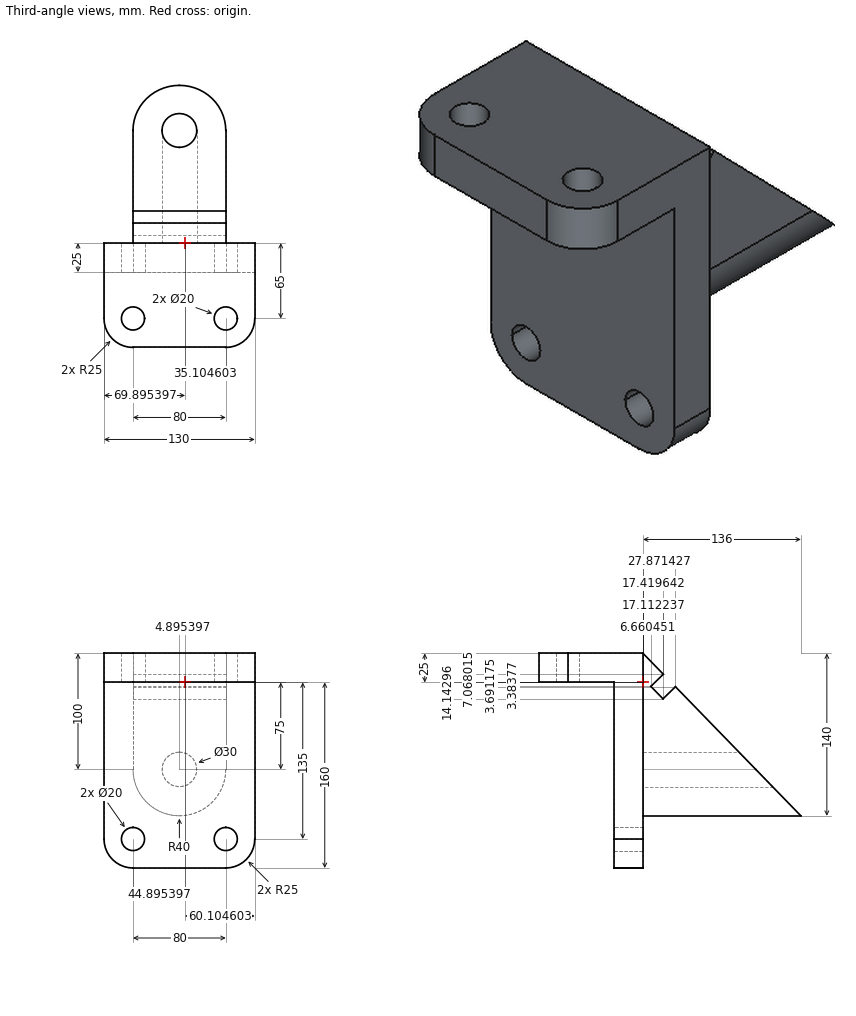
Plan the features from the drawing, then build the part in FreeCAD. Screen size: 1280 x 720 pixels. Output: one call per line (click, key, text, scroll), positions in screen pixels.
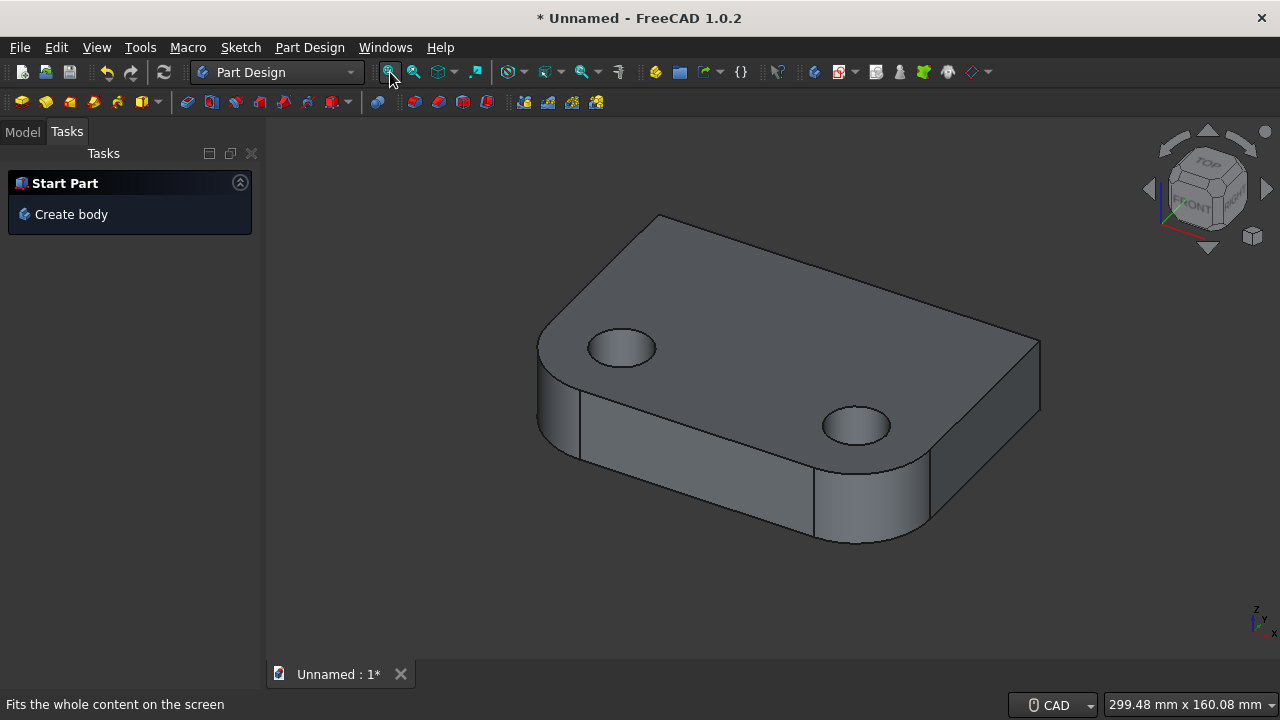
click(840, 72)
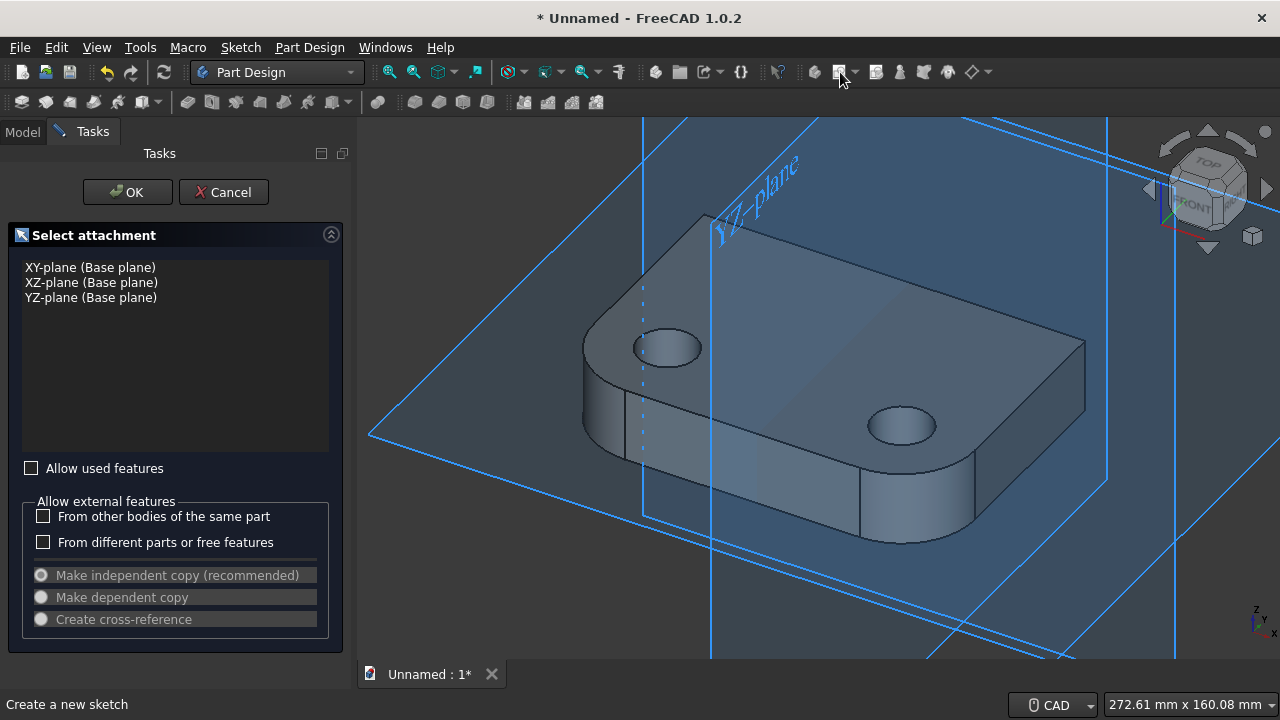
click(82, 268)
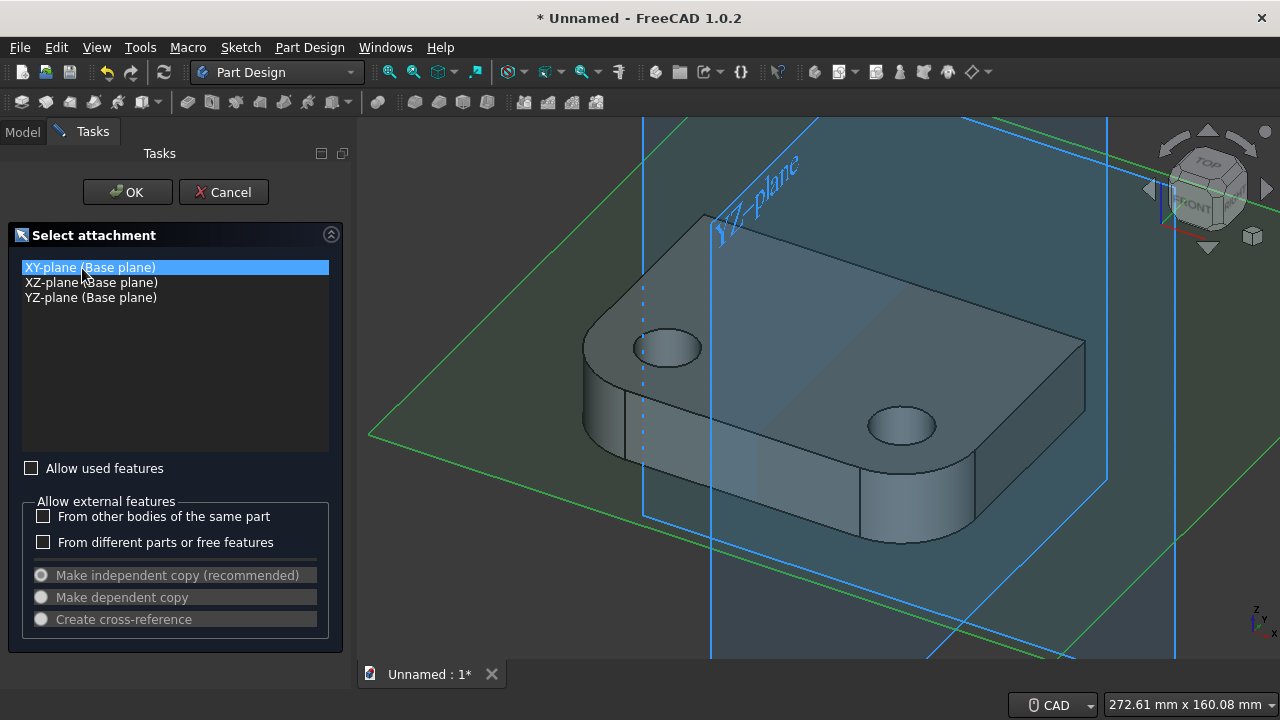
click(128, 192)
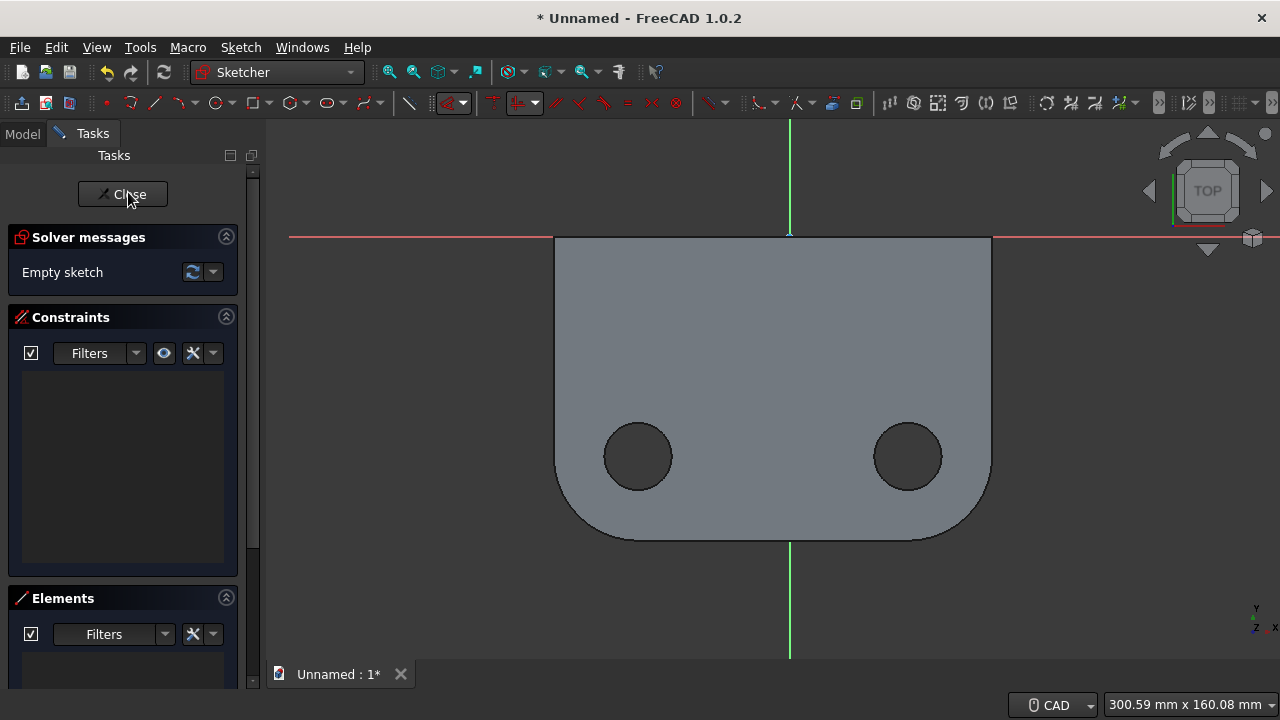
click(70, 104)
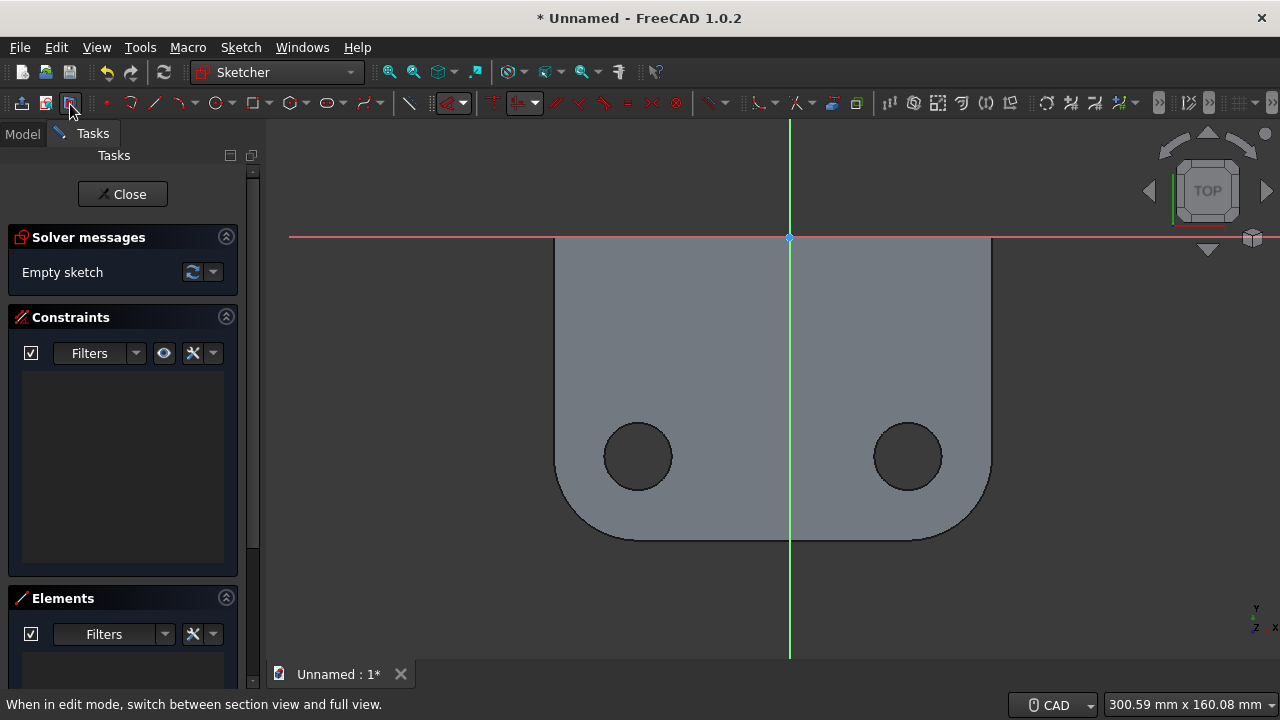
click(254, 104)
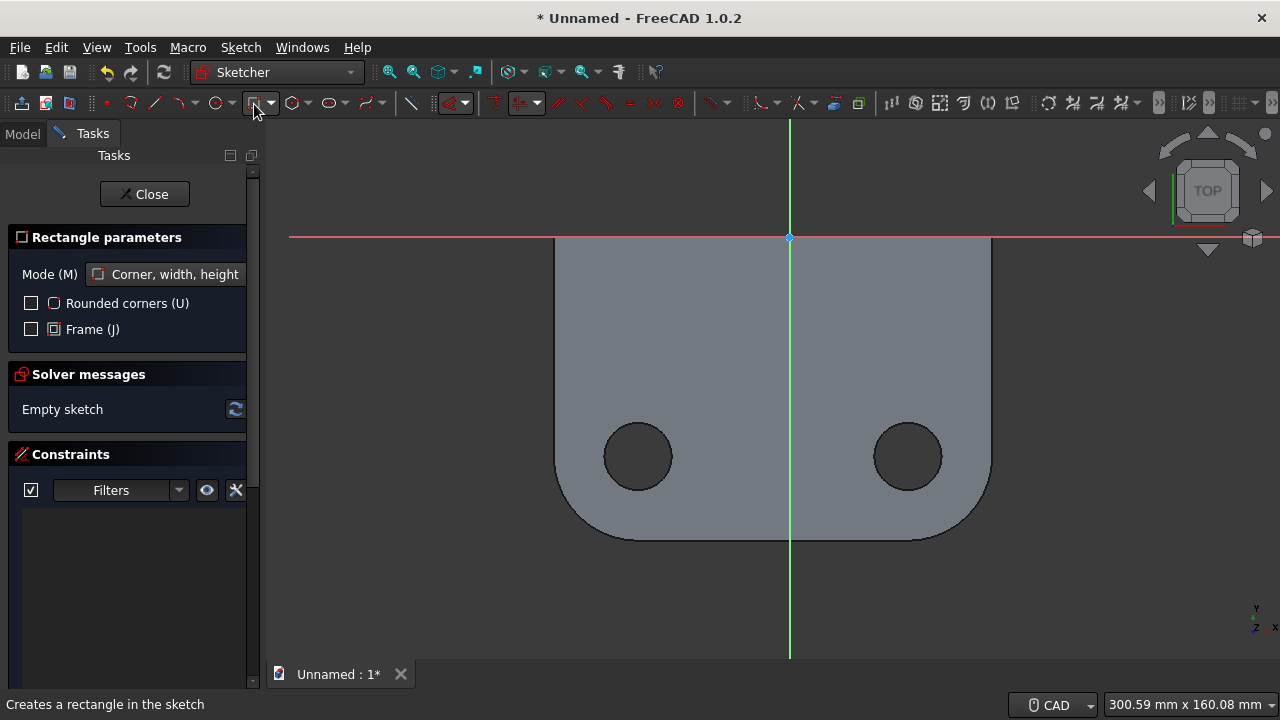
click(554, 237)
click(992, 322)
key(Escape)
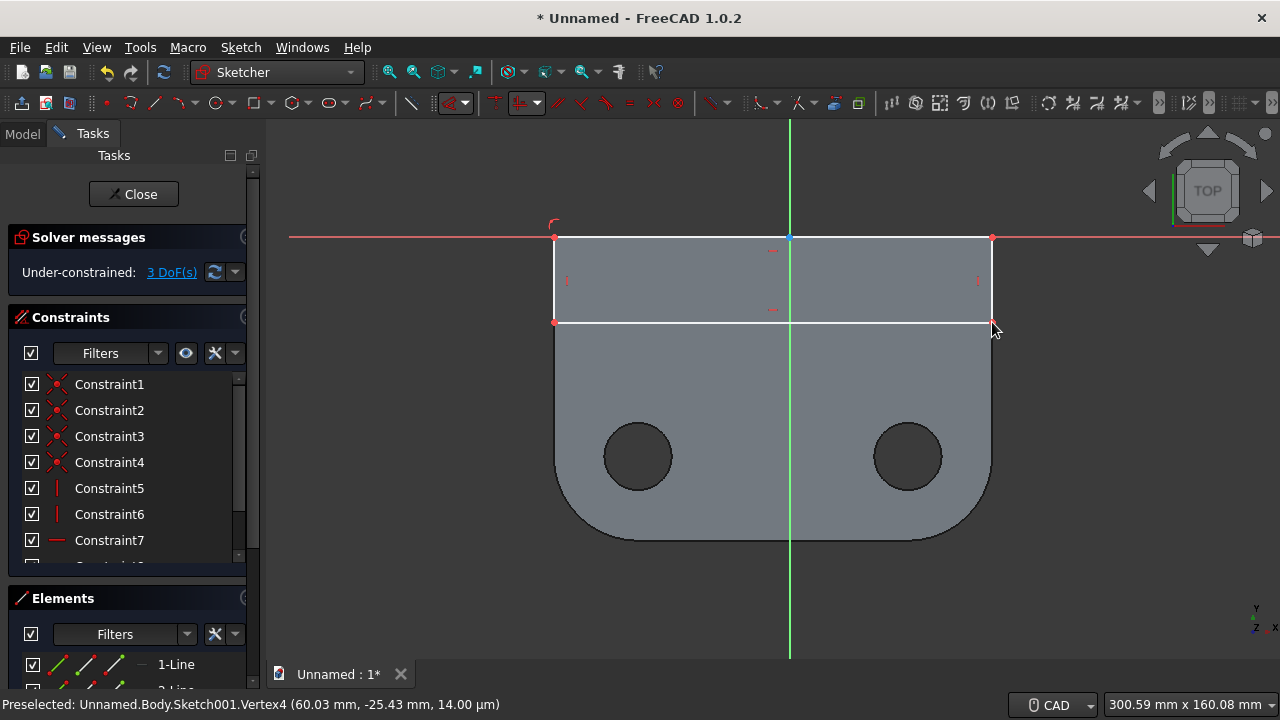
click(554, 263)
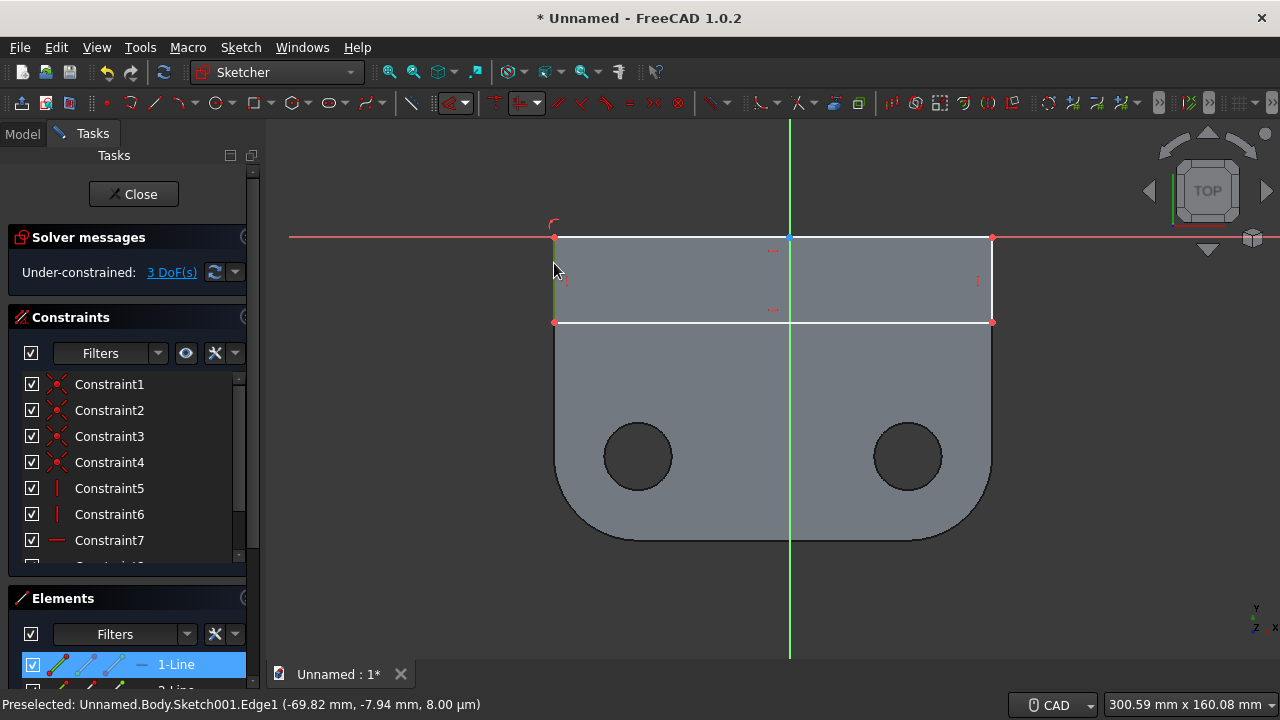
click(468, 104)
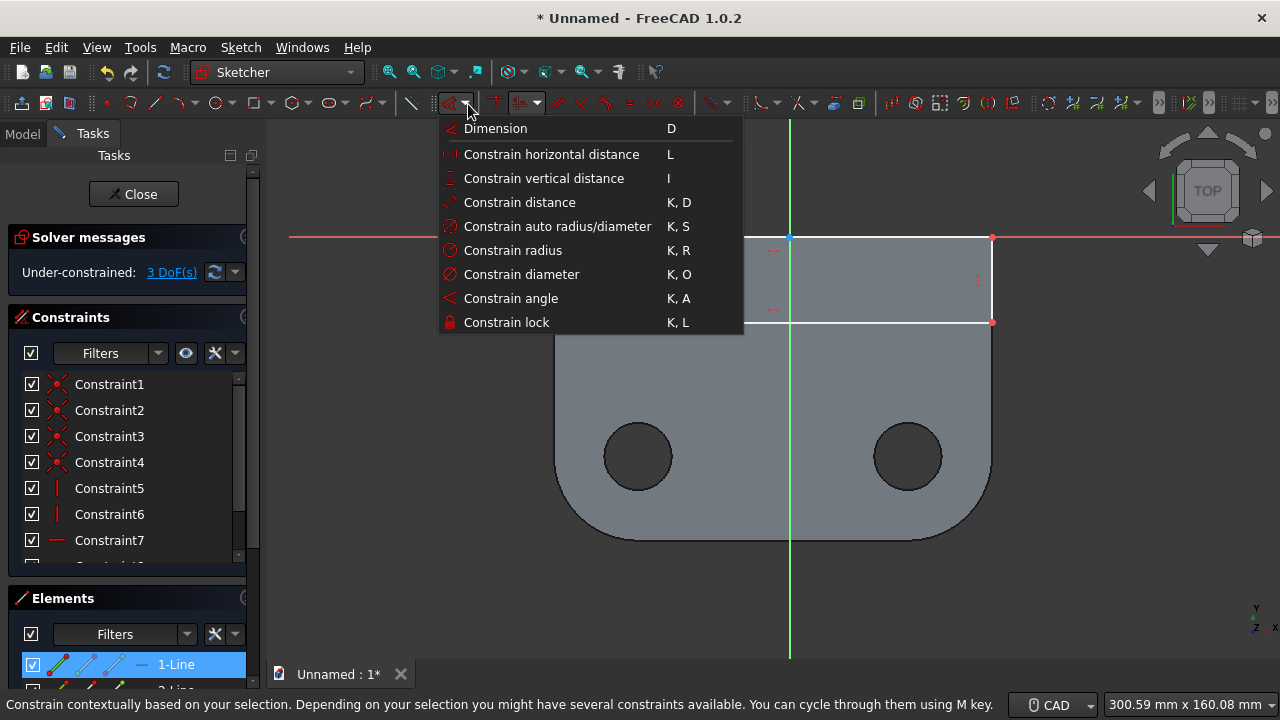
click(591, 178)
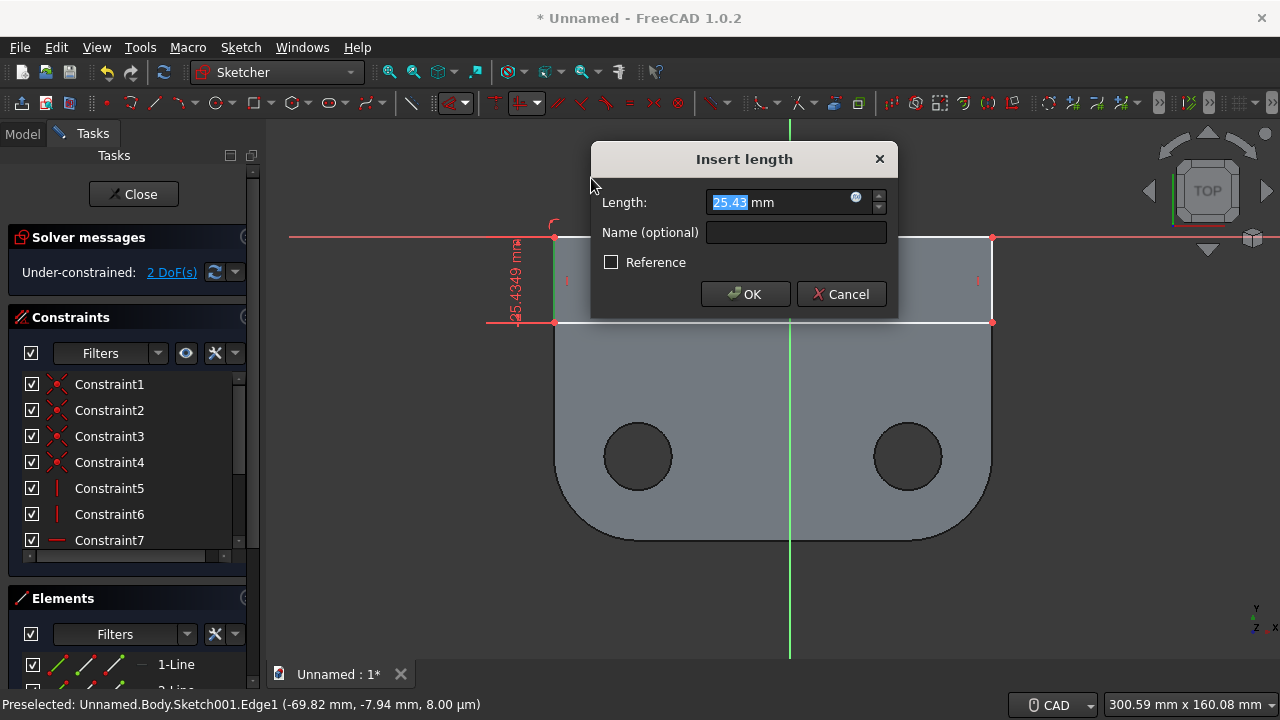
text(25)
key(Return)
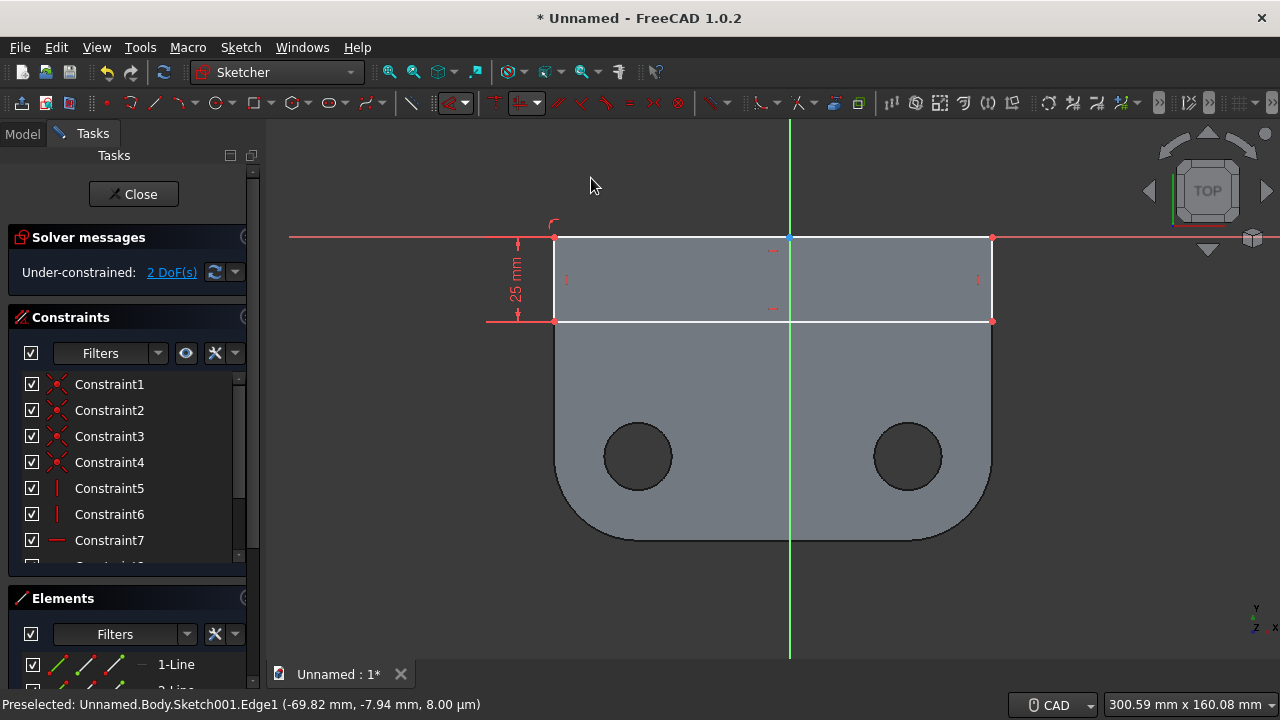
click(685, 322)